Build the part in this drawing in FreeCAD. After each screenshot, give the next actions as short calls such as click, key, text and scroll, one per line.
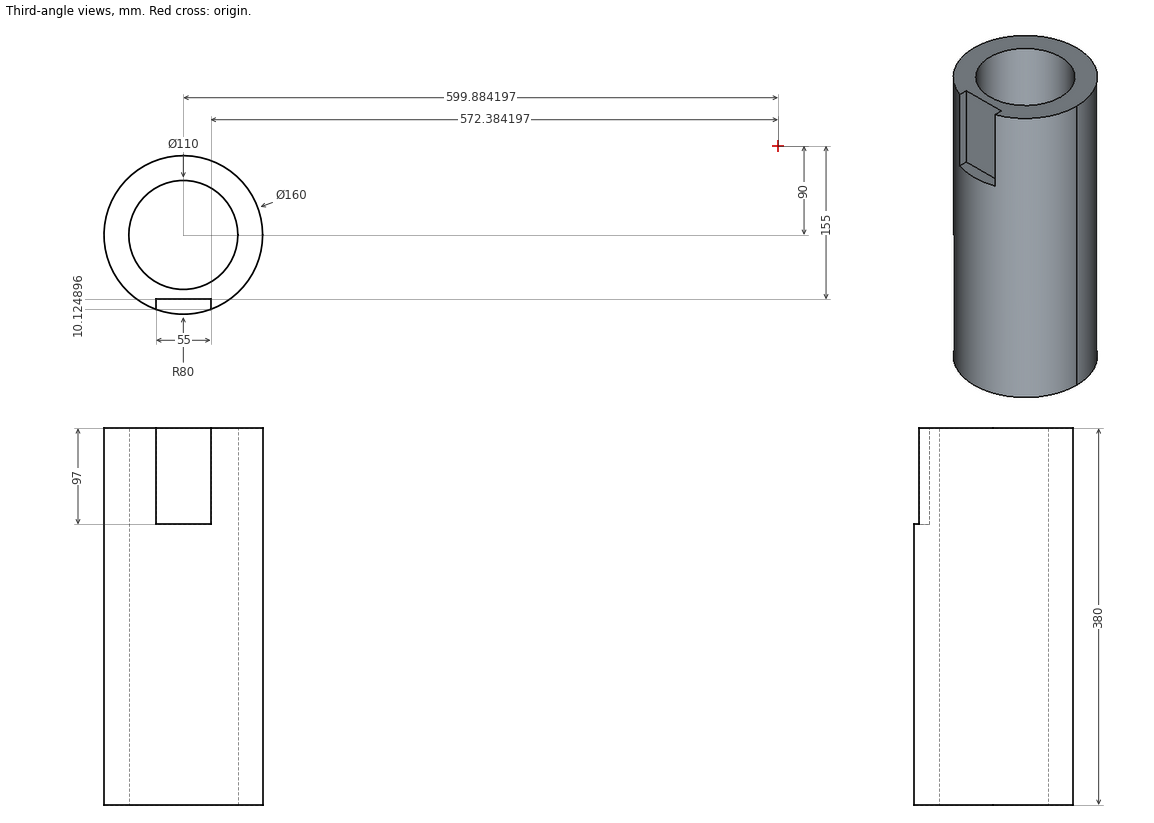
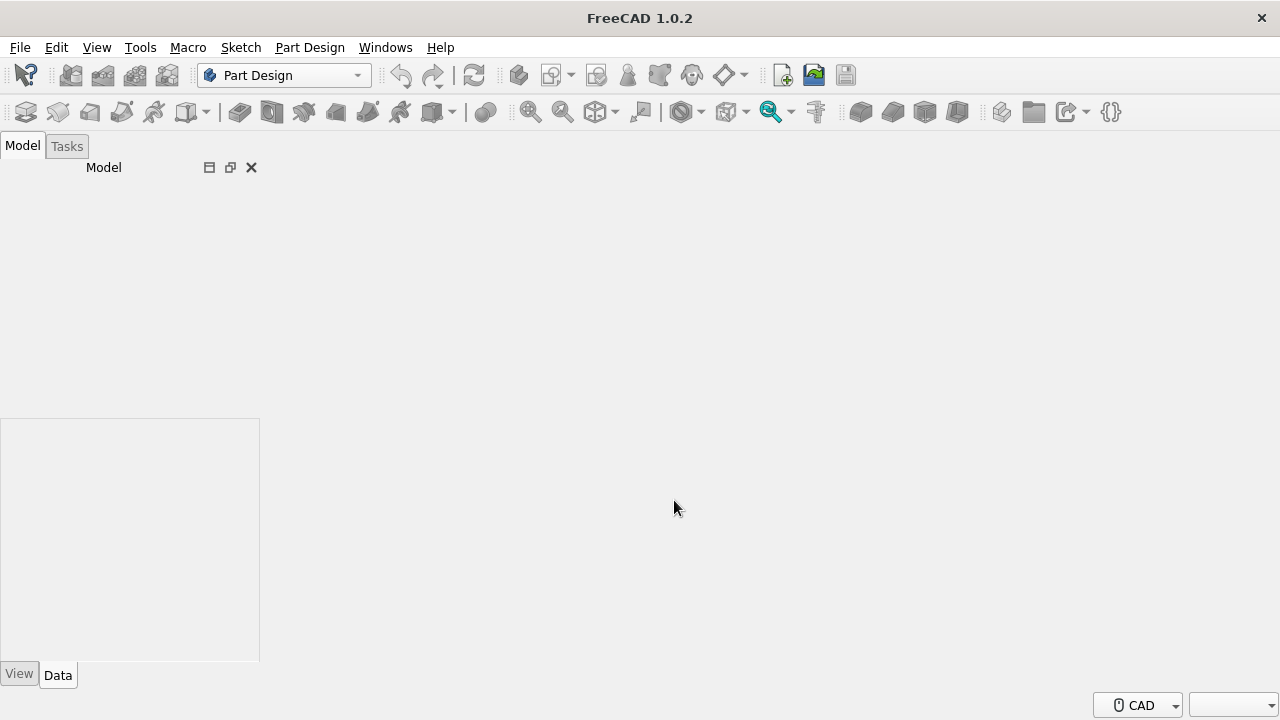
click(782, 76)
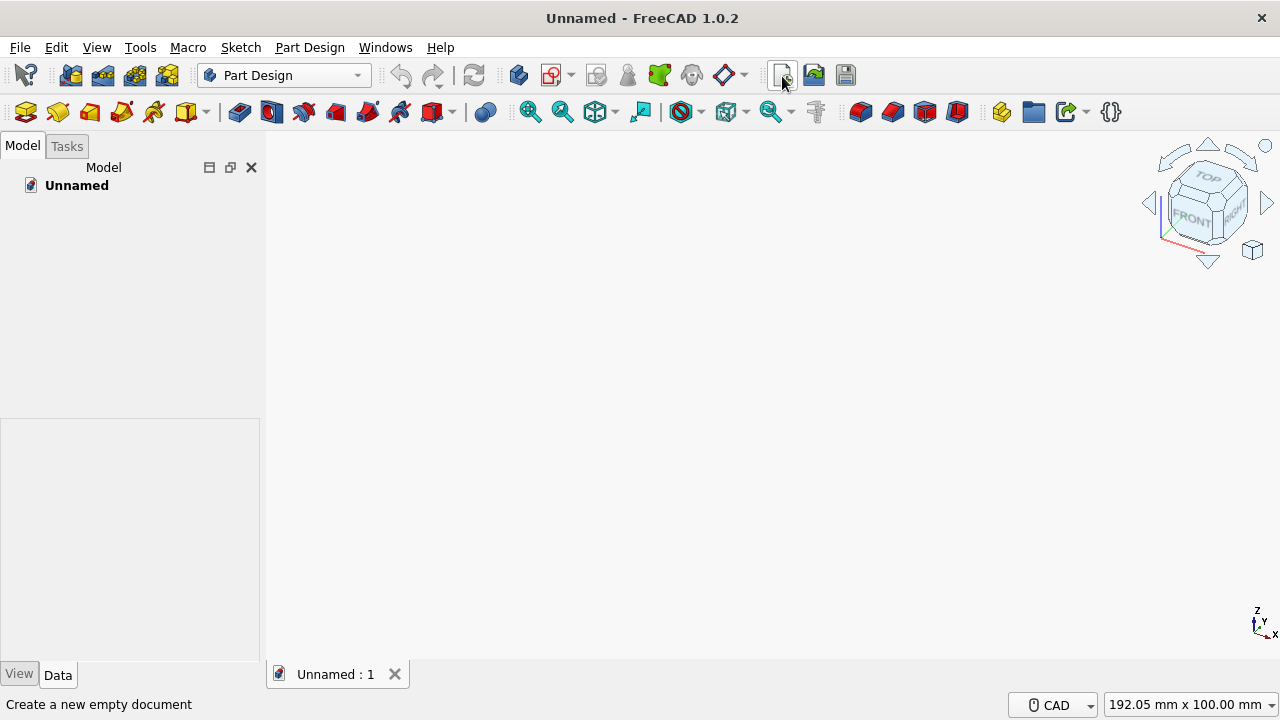
click(552, 76)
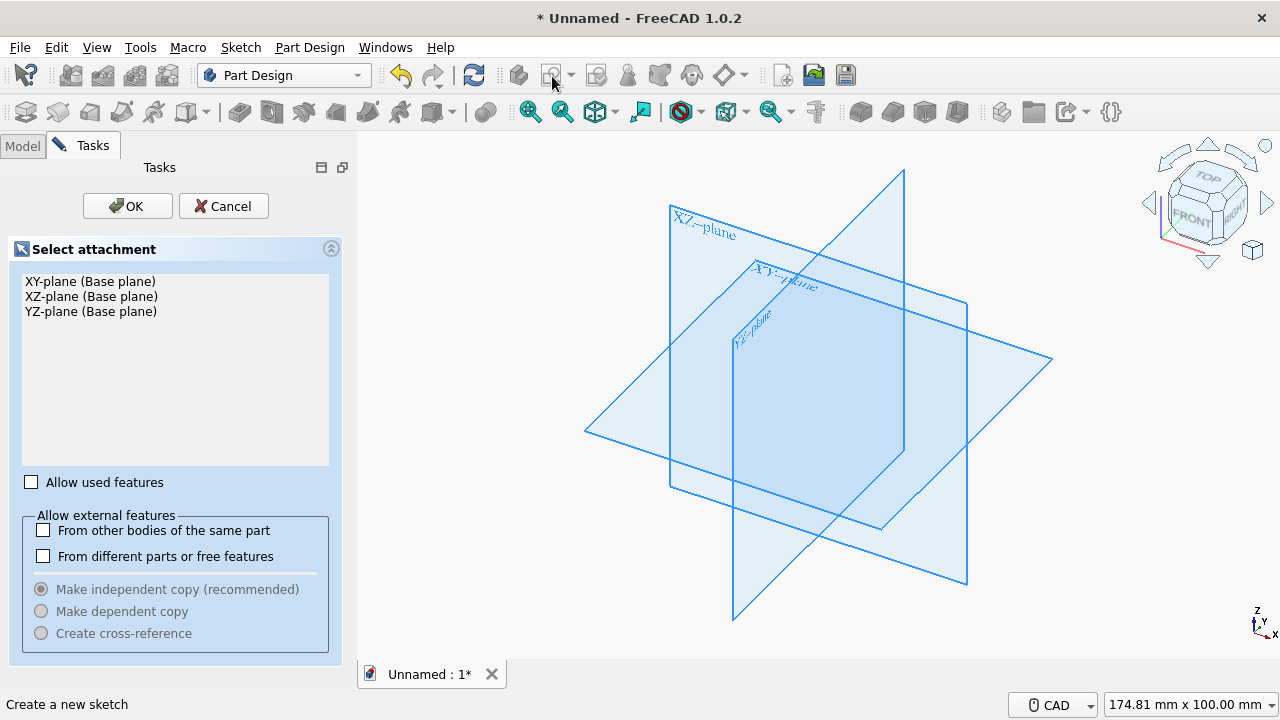
click(82, 282)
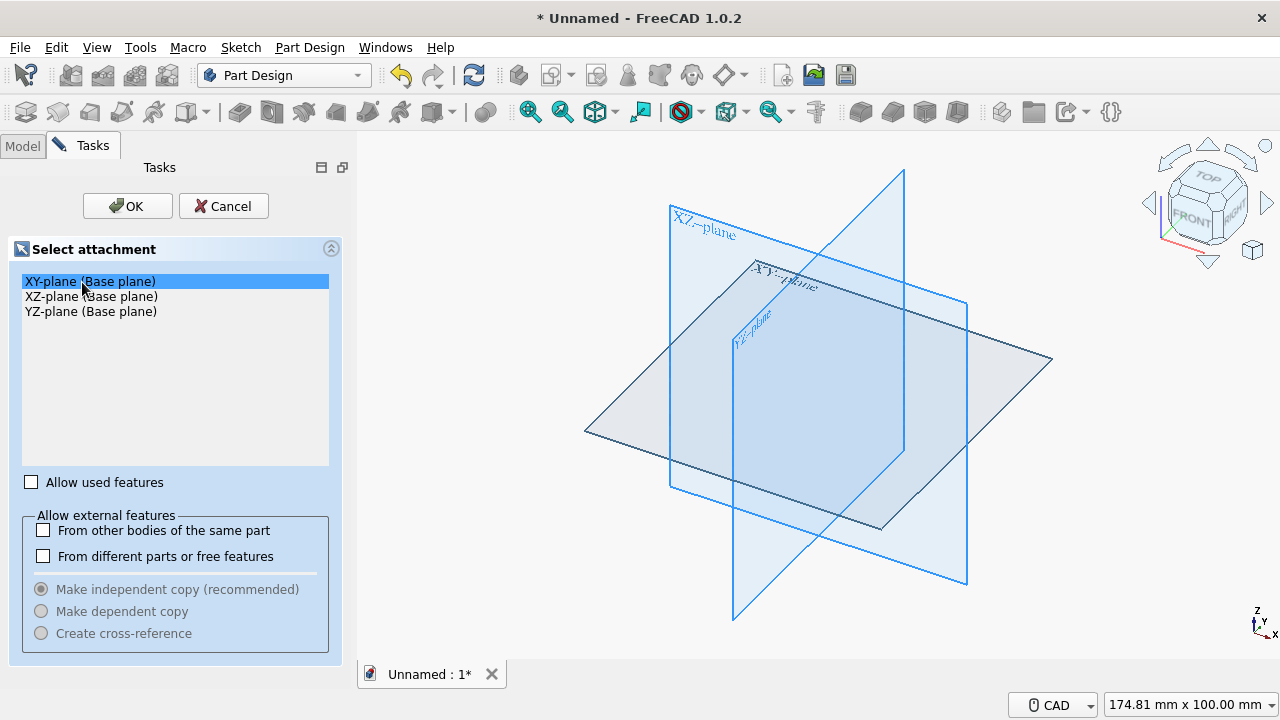
click(128, 206)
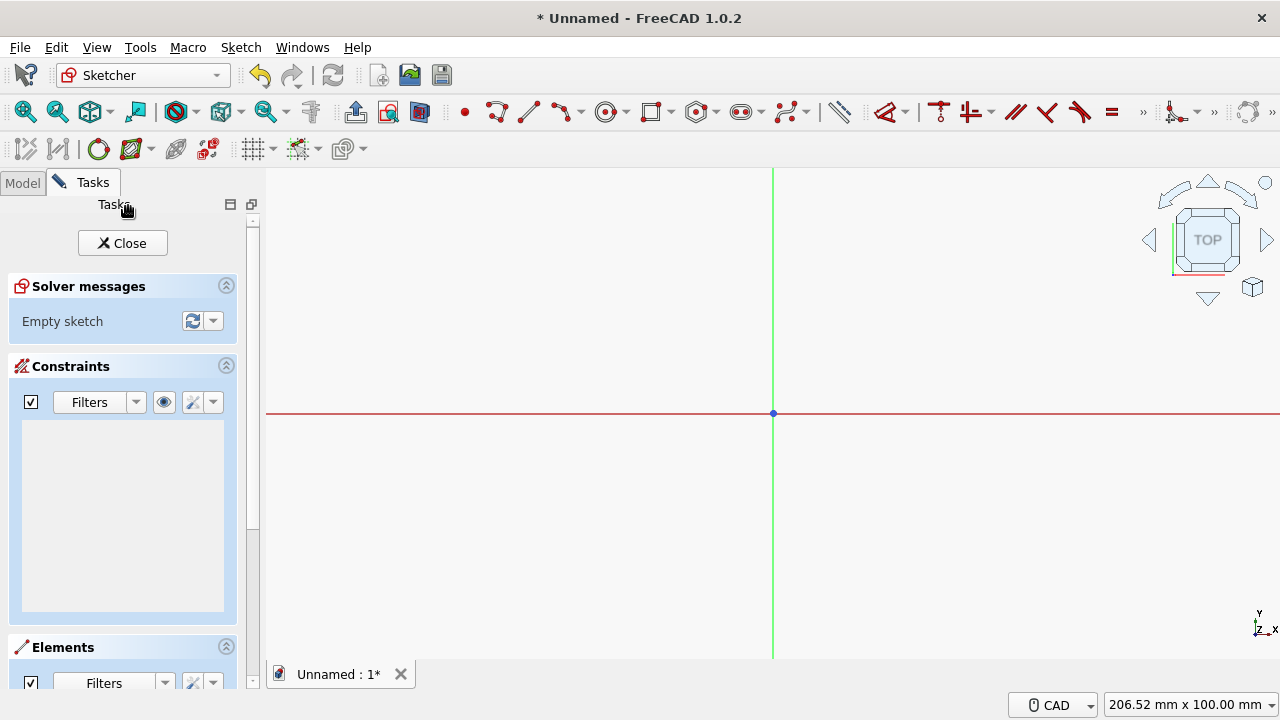
scroll(1115, 302, down, 8)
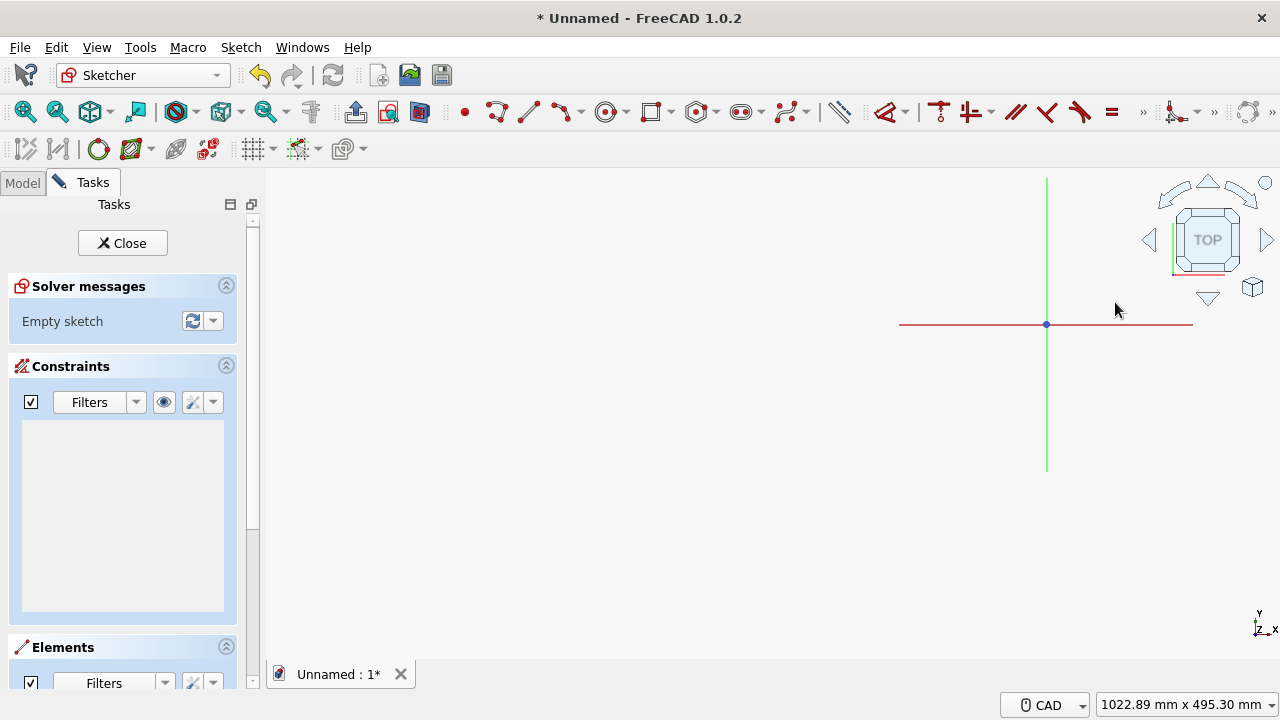
scroll(294, 414, up, 3)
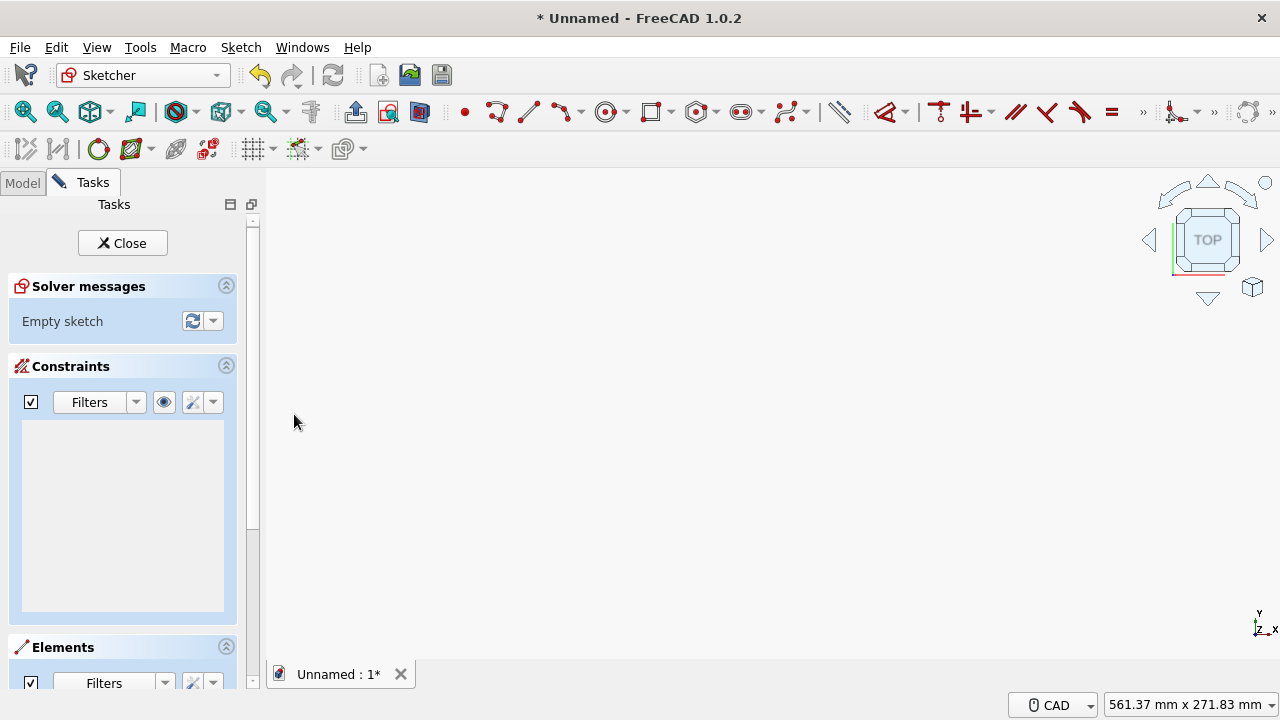
click(606, 112)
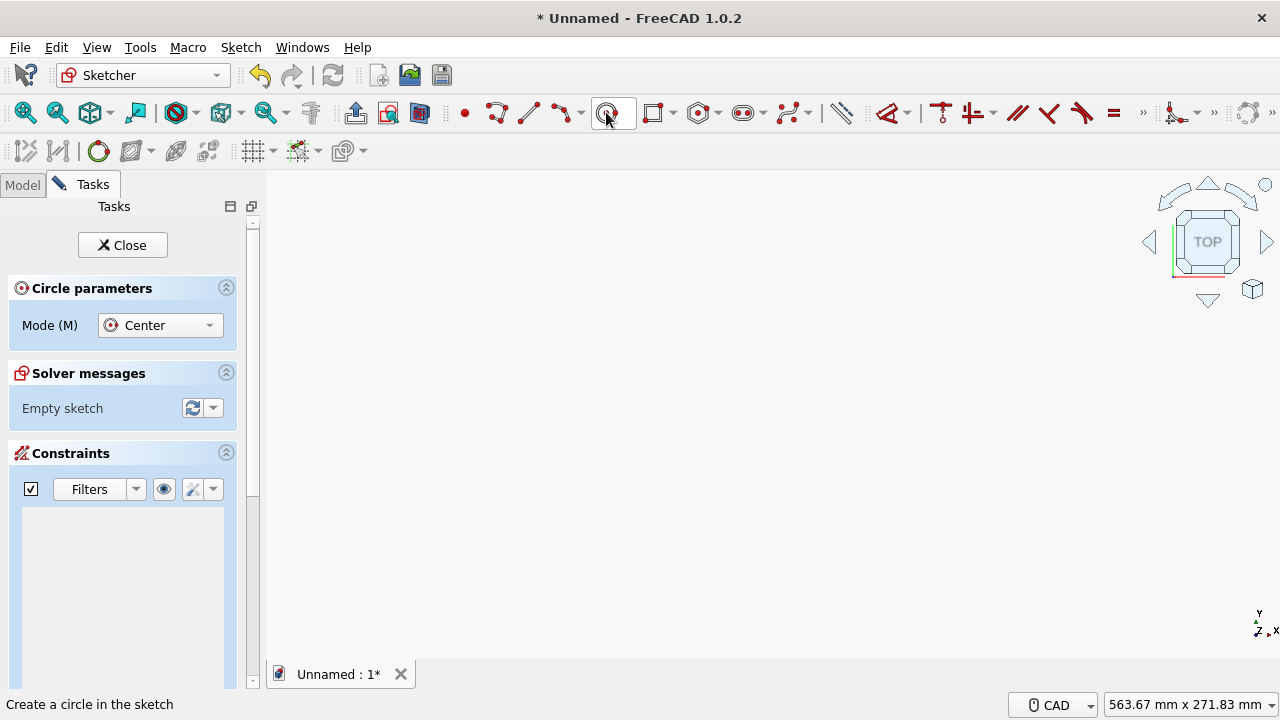
click(583, 414)
click(684, 313)
key(Escape)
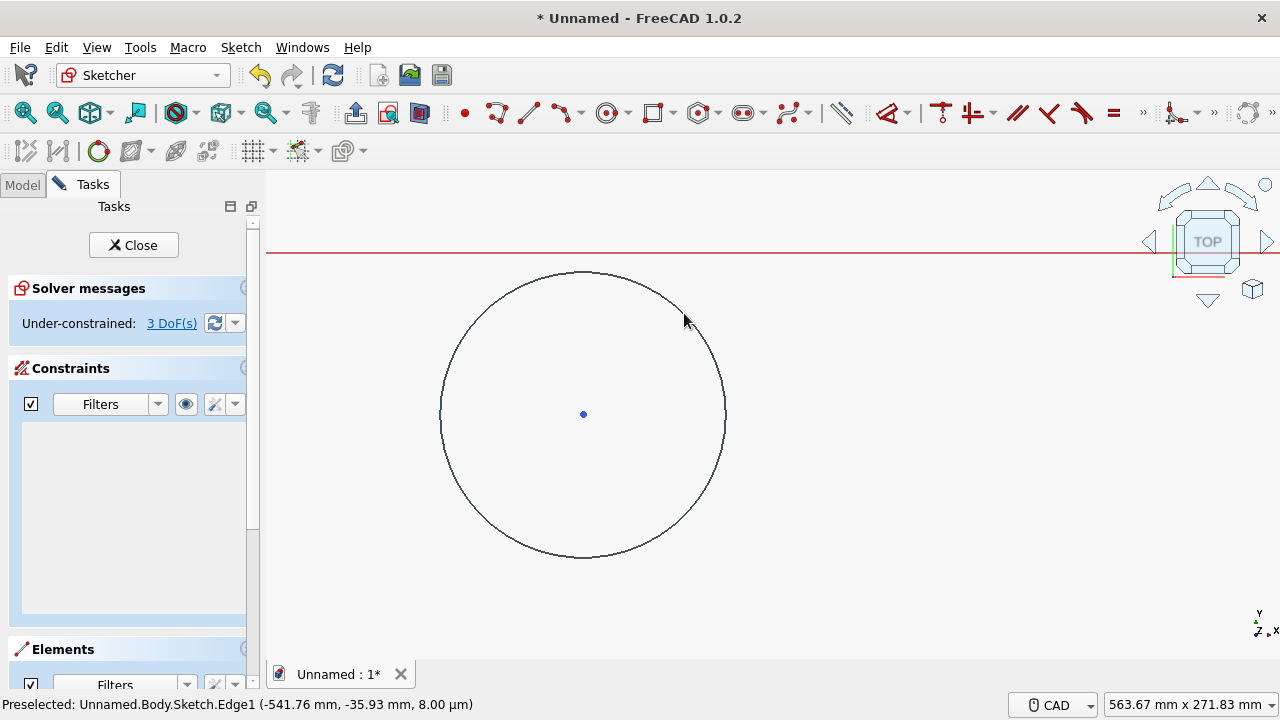
click(888, 114)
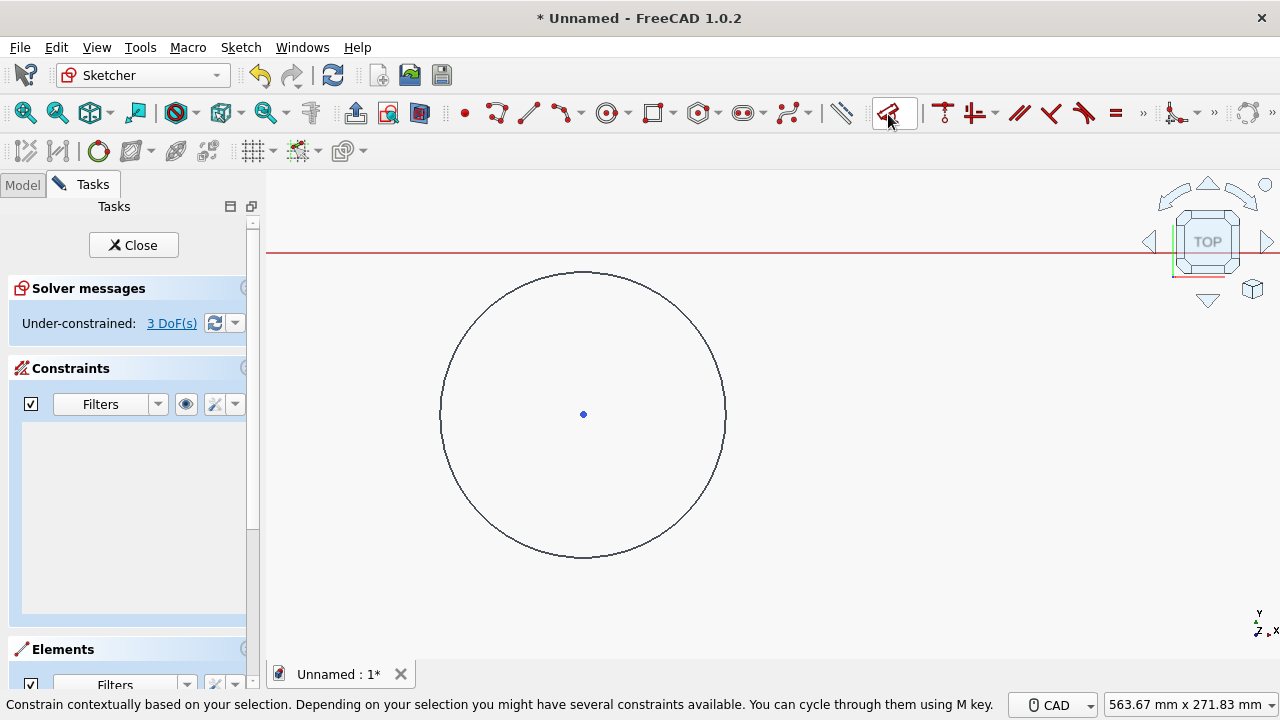
click(684, 314)
click(707, 291)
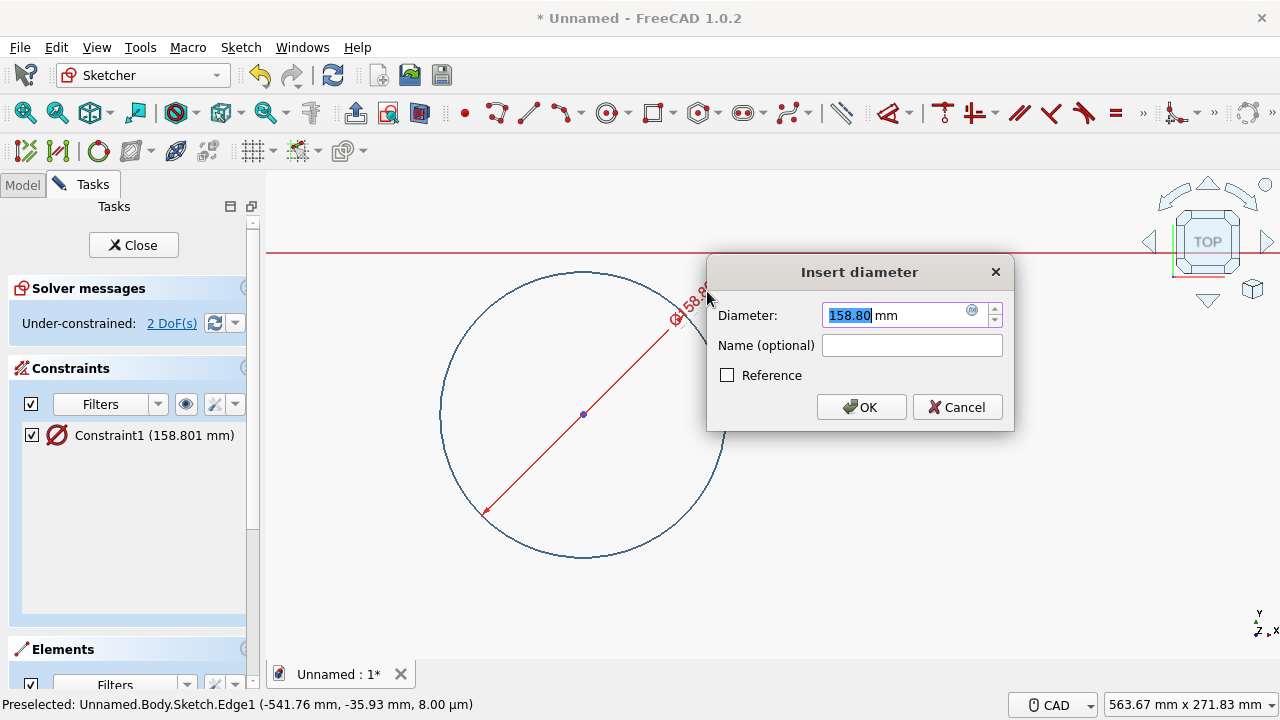
text(160)
key(Return)